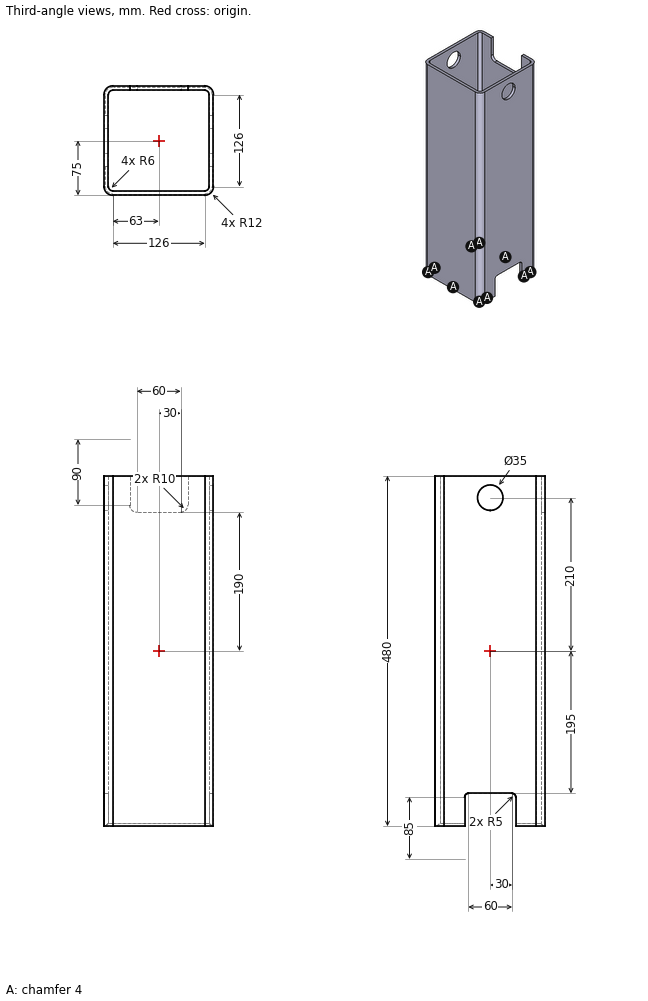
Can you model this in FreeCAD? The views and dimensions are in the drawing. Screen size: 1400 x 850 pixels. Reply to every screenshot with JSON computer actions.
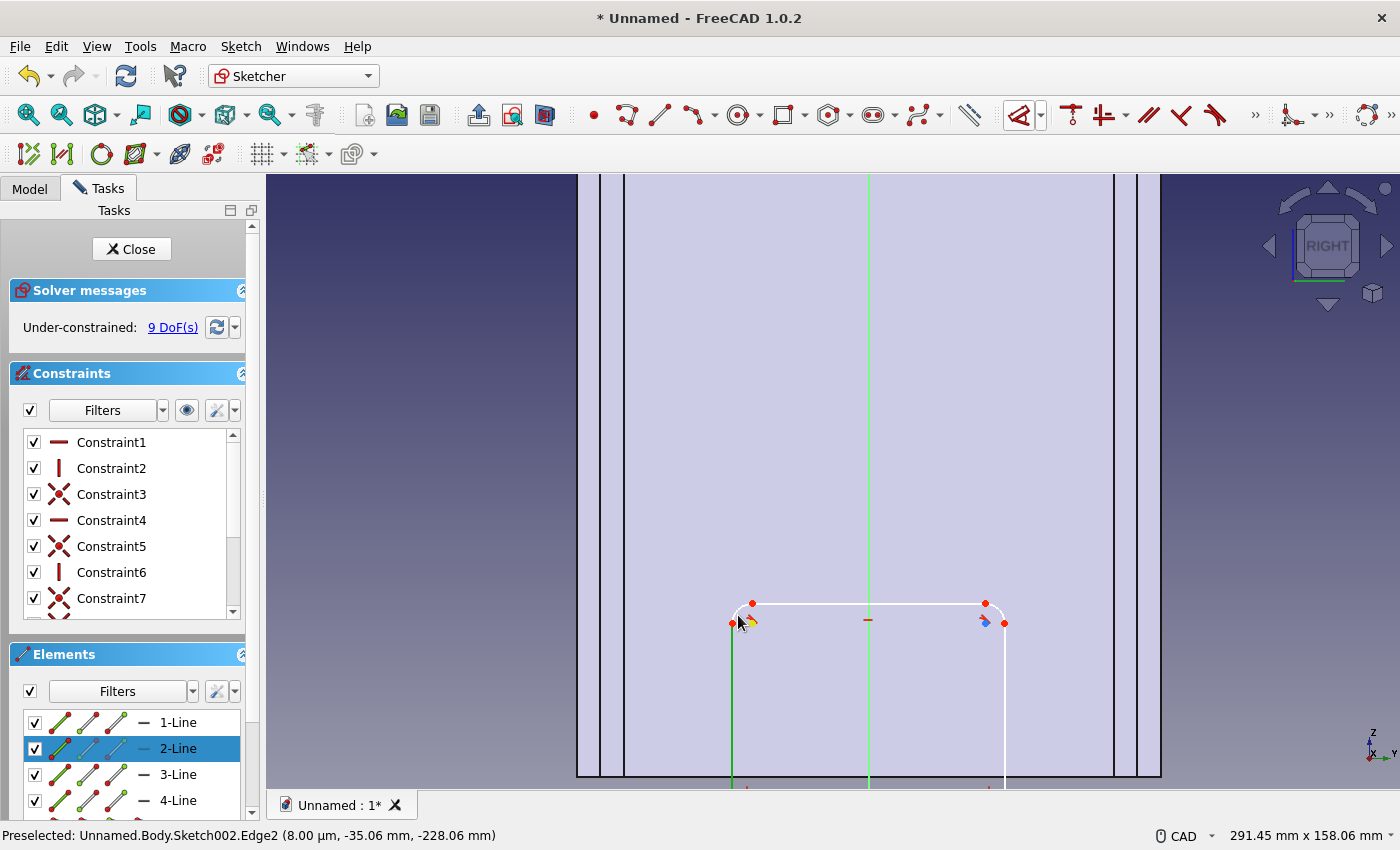
{"action": "left_click", "coordinate": [738, 610]}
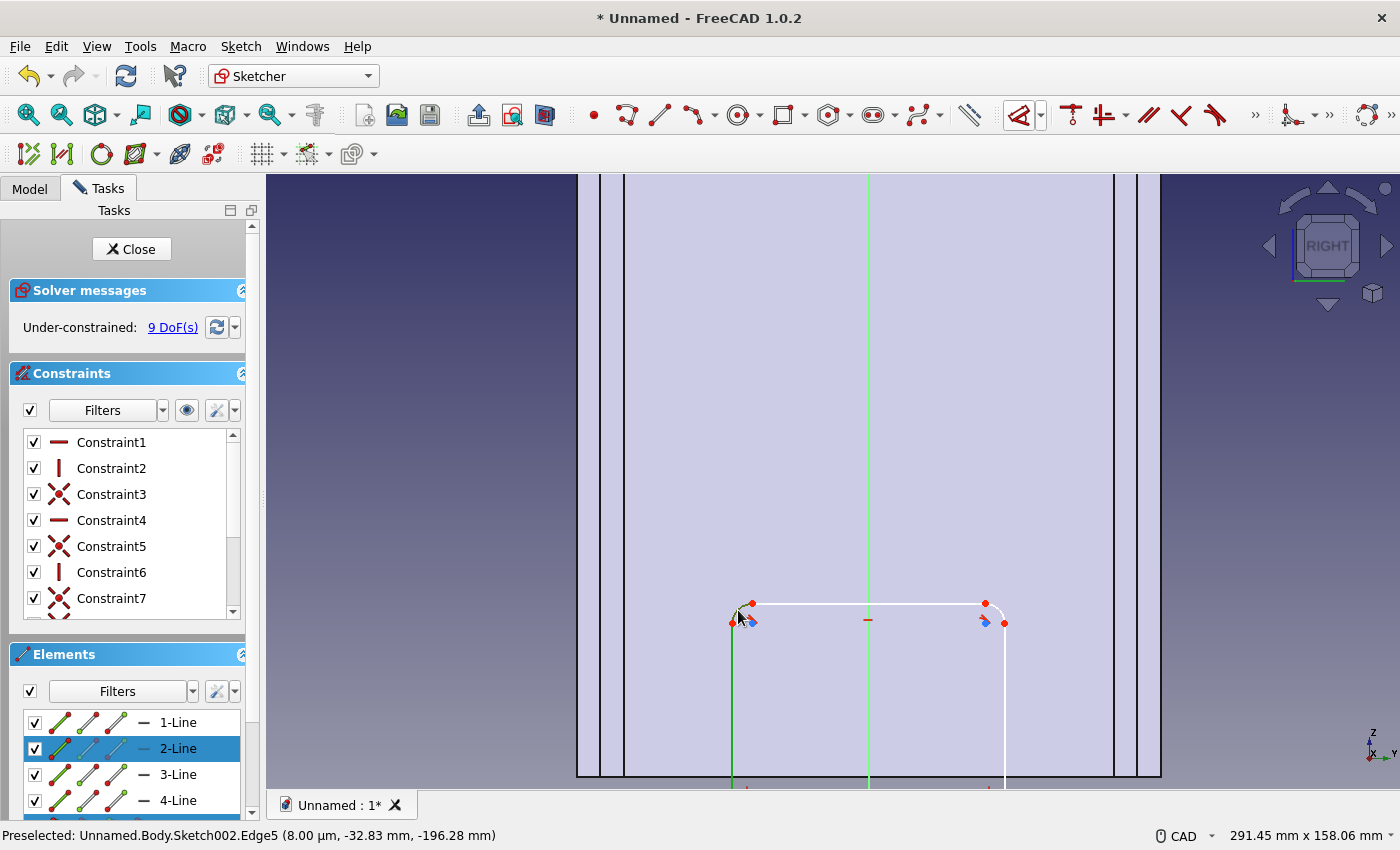
{"action": "key", "text": "t"}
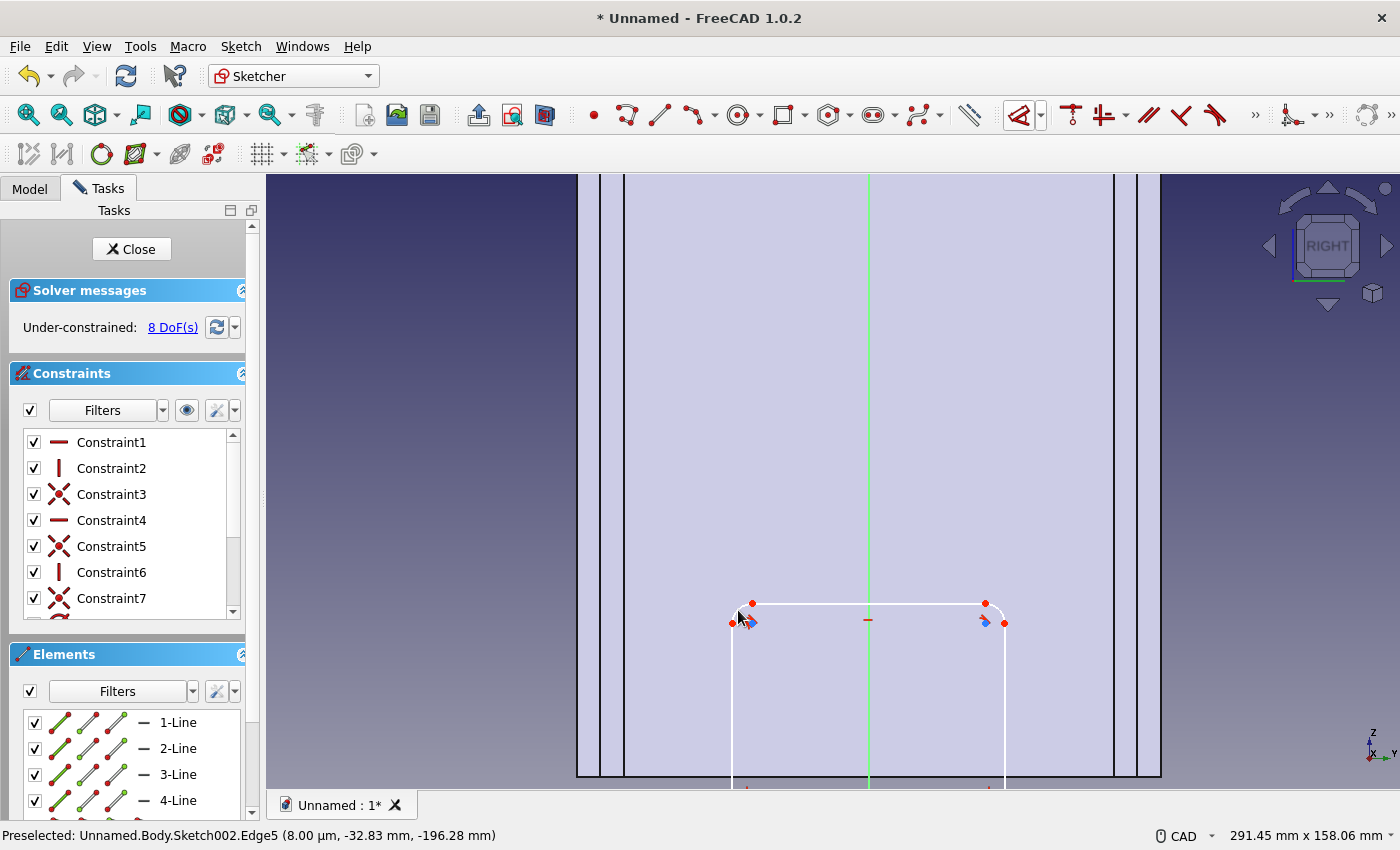
{"action": "scroll", "coordinate": [738, 615], "scroll_direction": "down", "scroll_amount": 8}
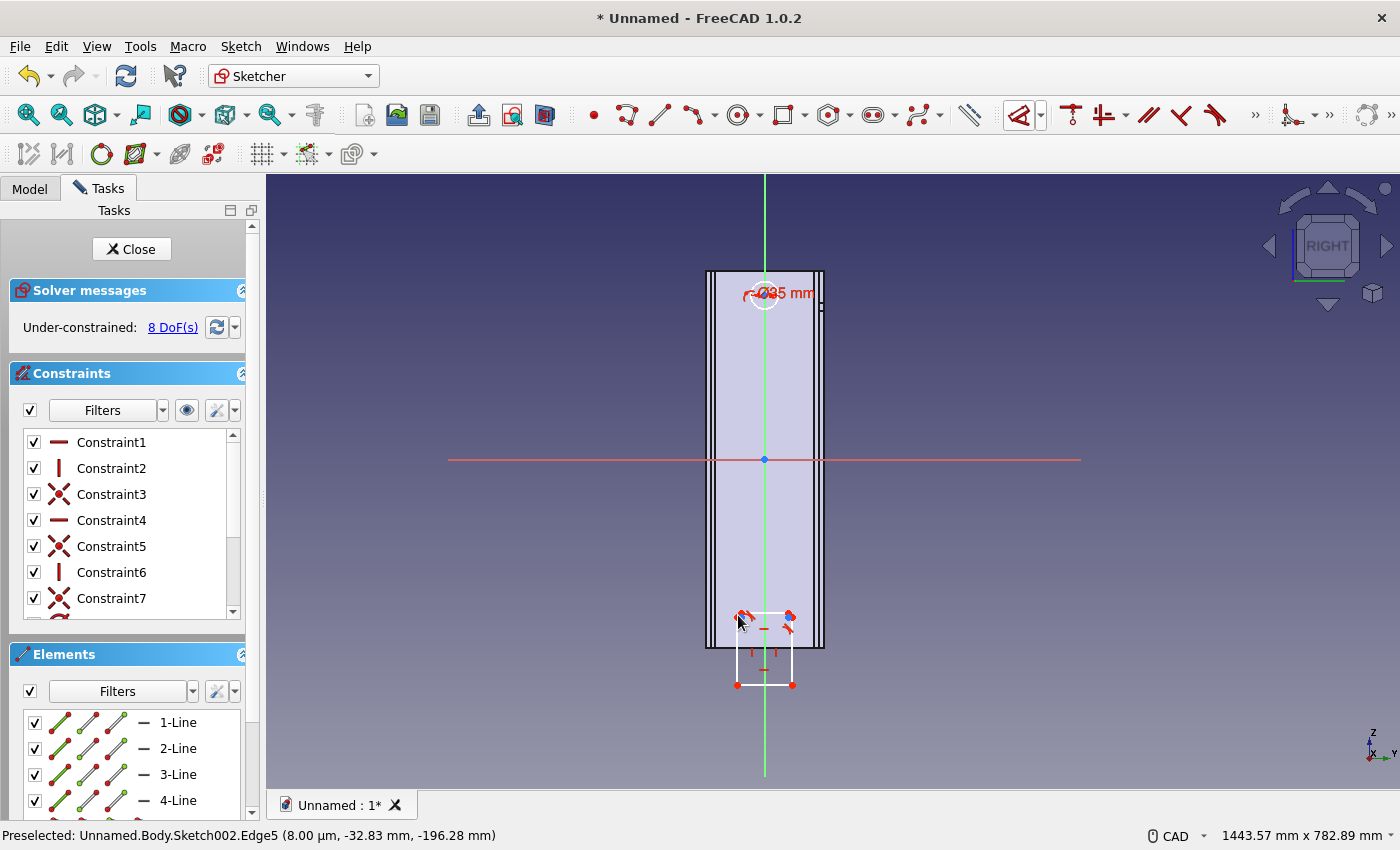
{"action": "left_click", "coordinate": [792, 638]}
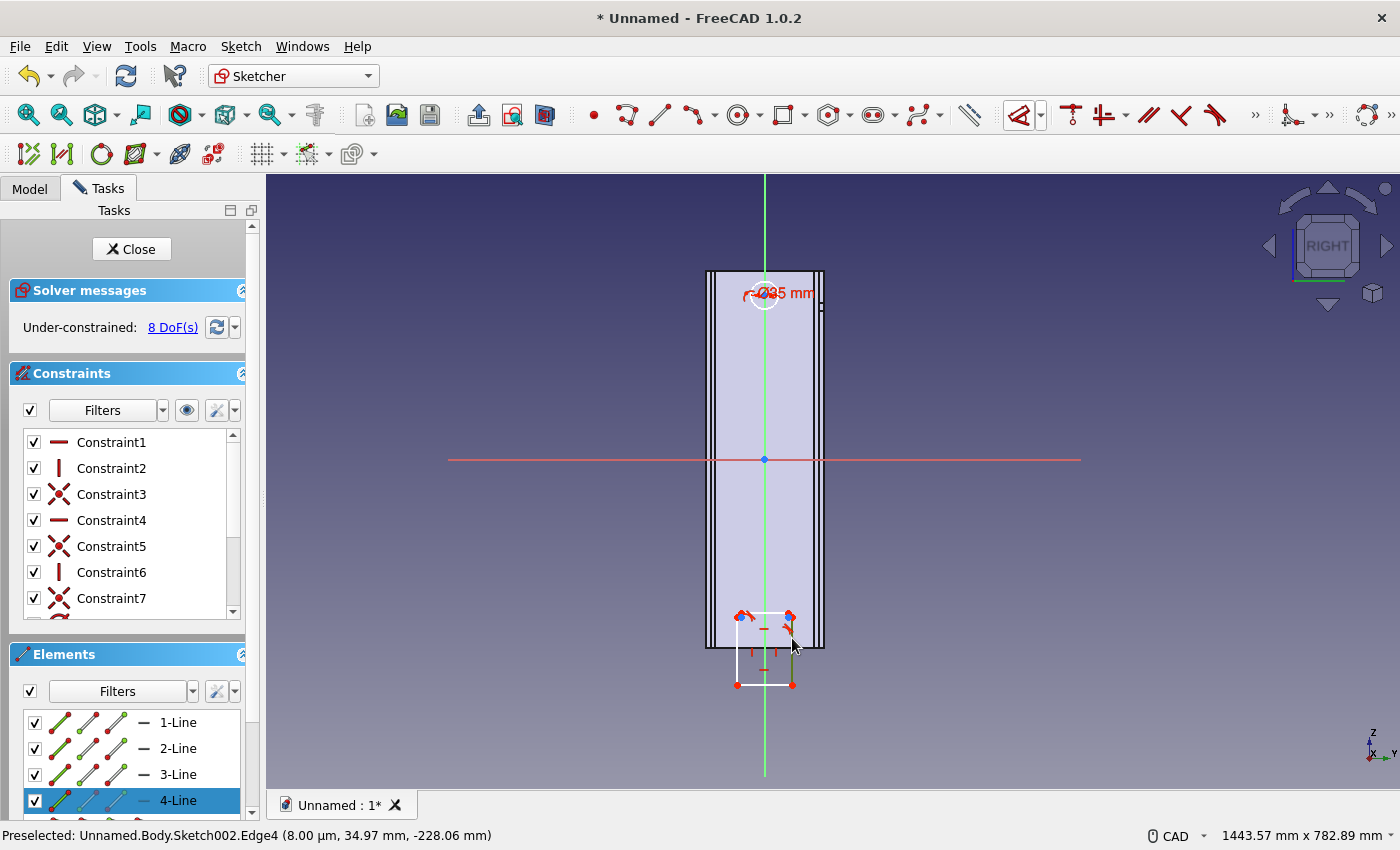
{"action": "scroll", "coordinate": [791, 615], "scroll_direction": "up", "scroll_amount": 8}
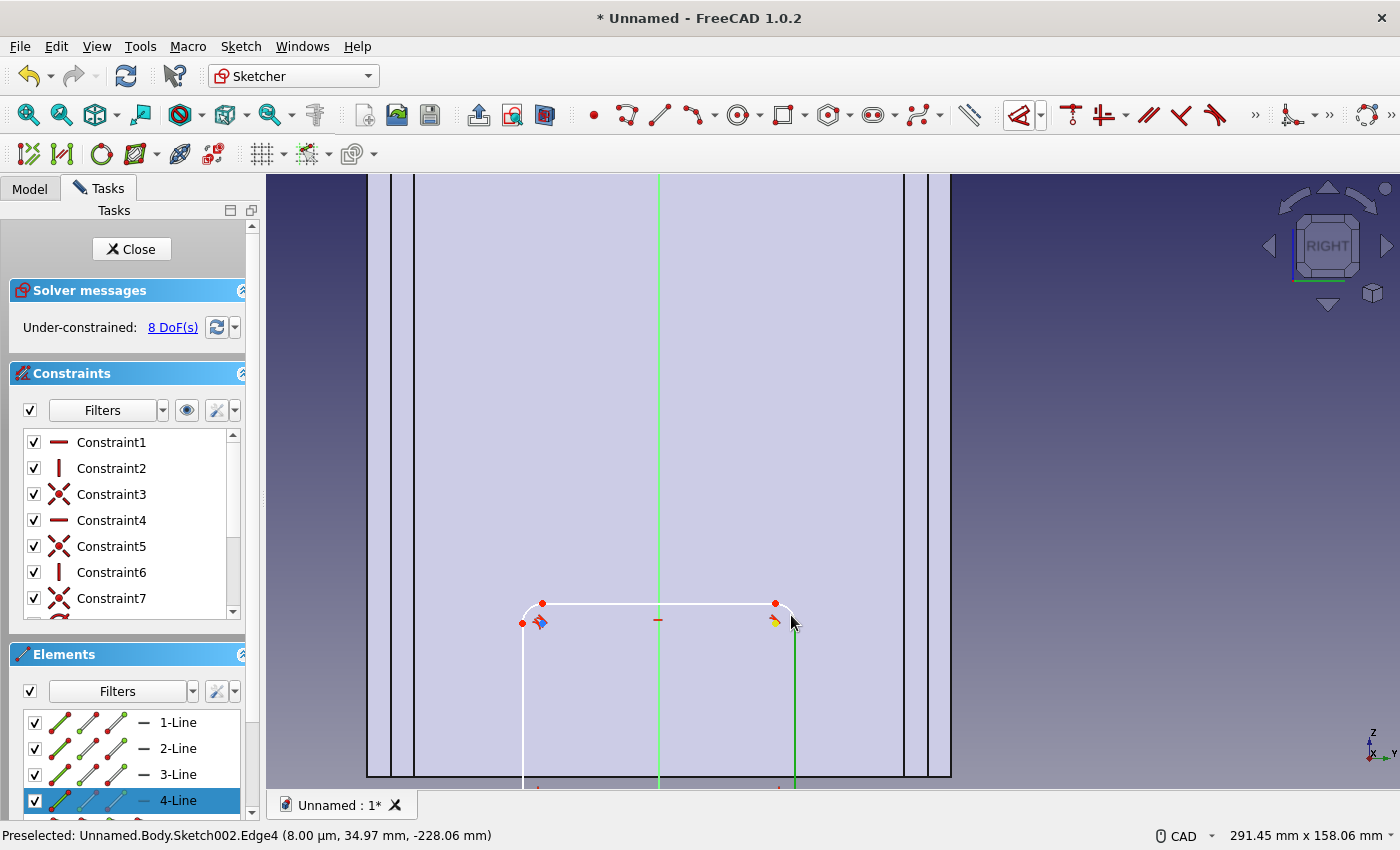
{"action": "left_click", "coordinate": [789, 610]}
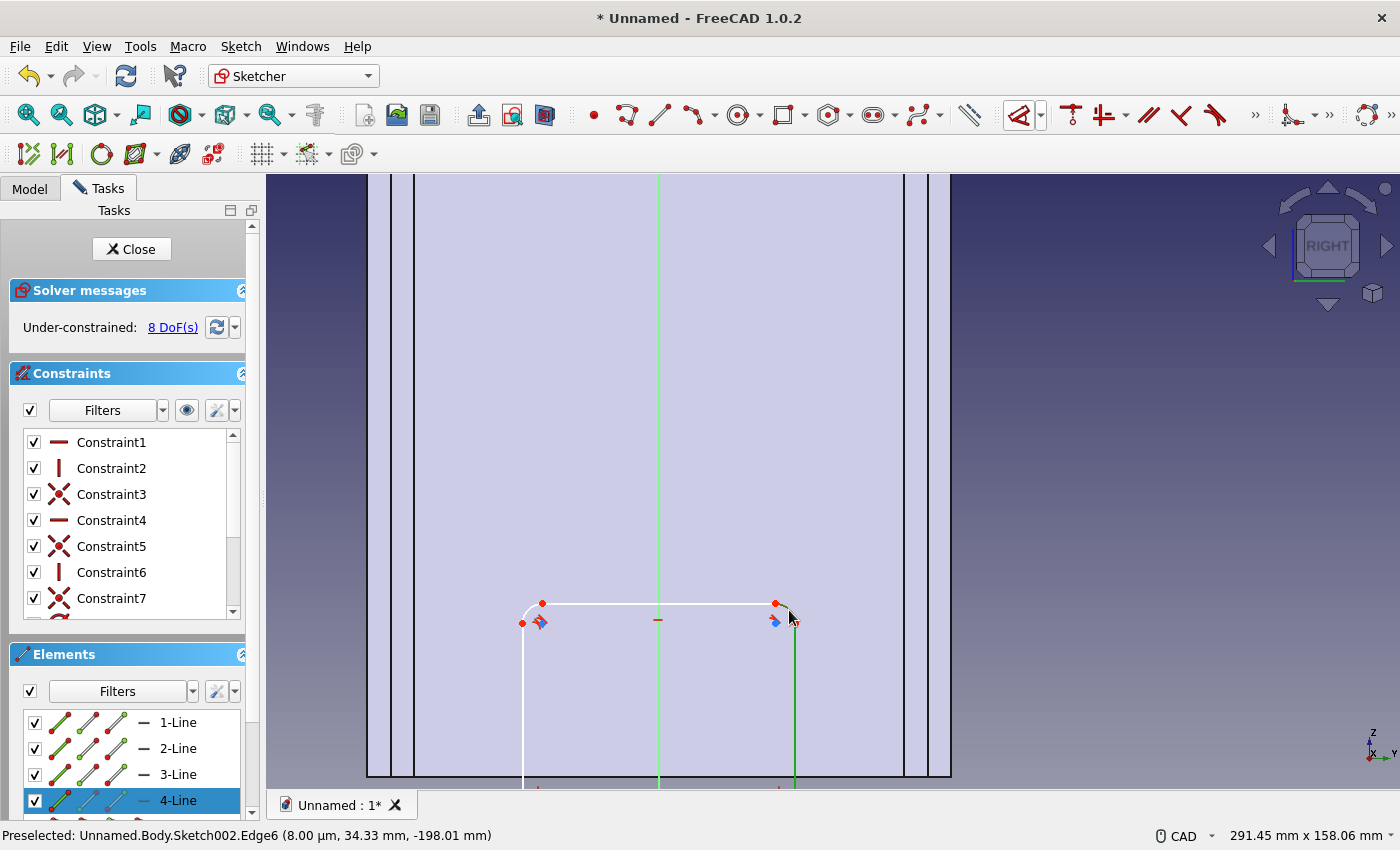
{"action": "key", "text": "t"}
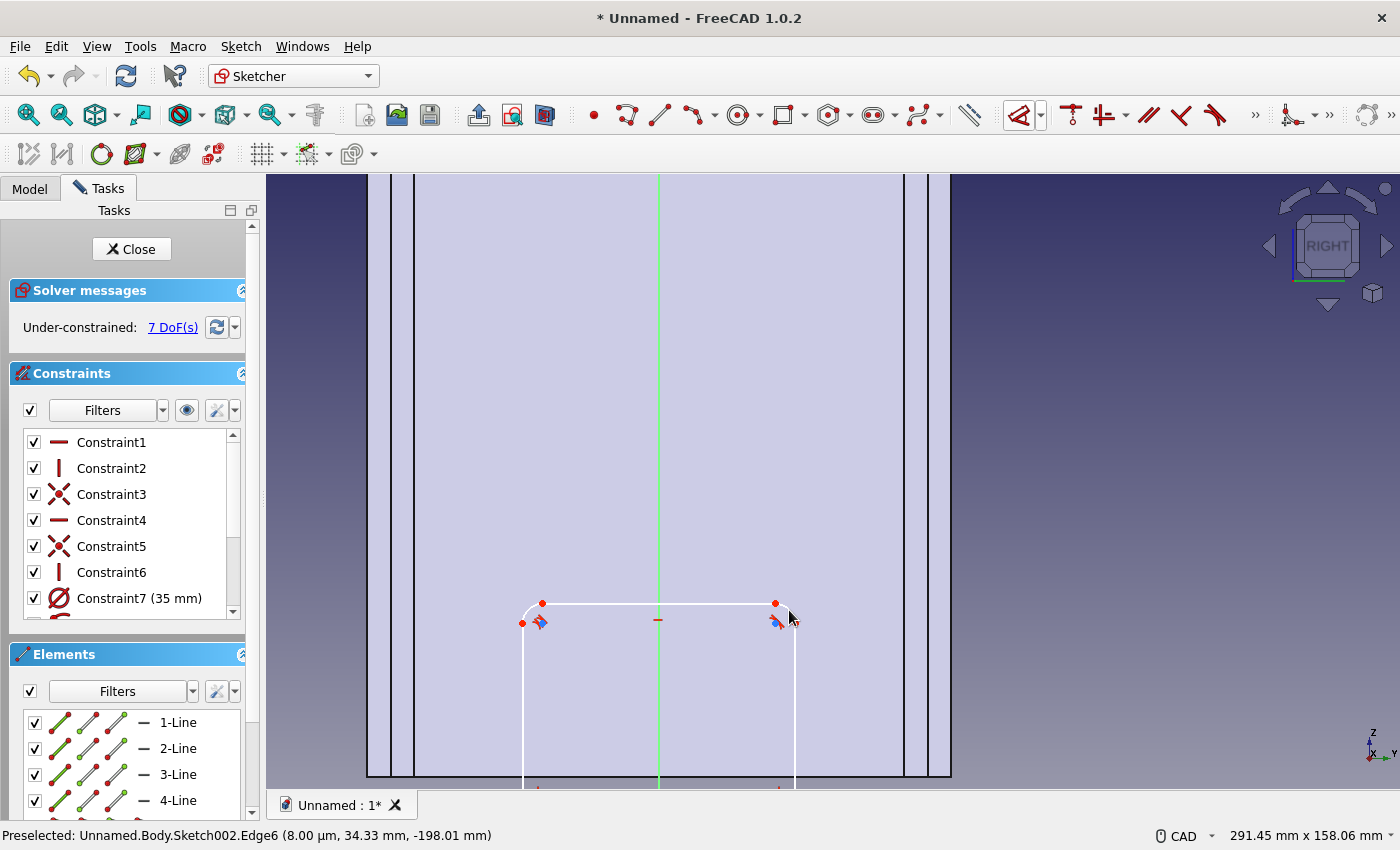
{"action": "scroll", "coordinate": [534, 606], "scroll_direction": "up", "scroll_amount": 2}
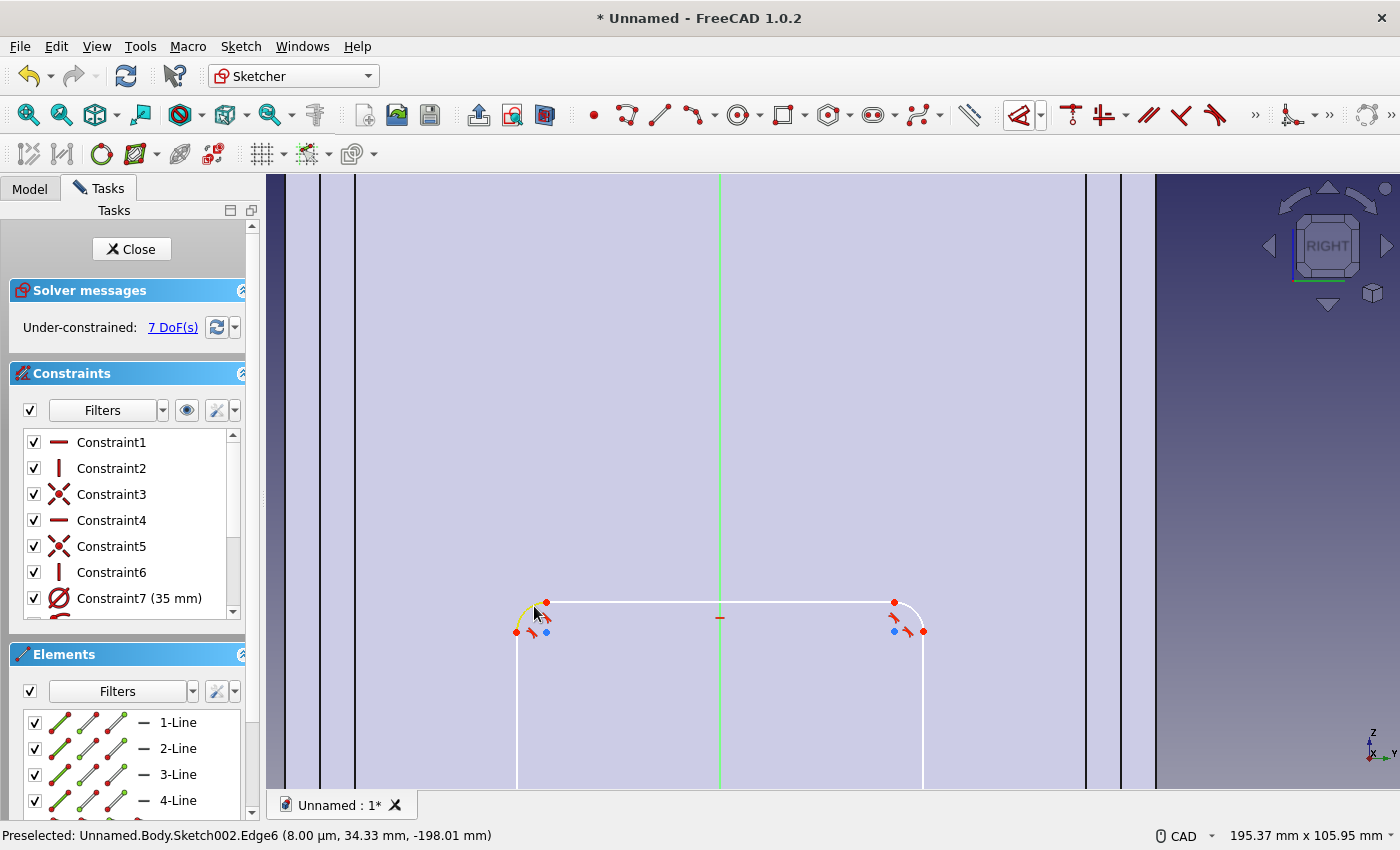
{"action": "left_click", "coordinate": [533, 606]}